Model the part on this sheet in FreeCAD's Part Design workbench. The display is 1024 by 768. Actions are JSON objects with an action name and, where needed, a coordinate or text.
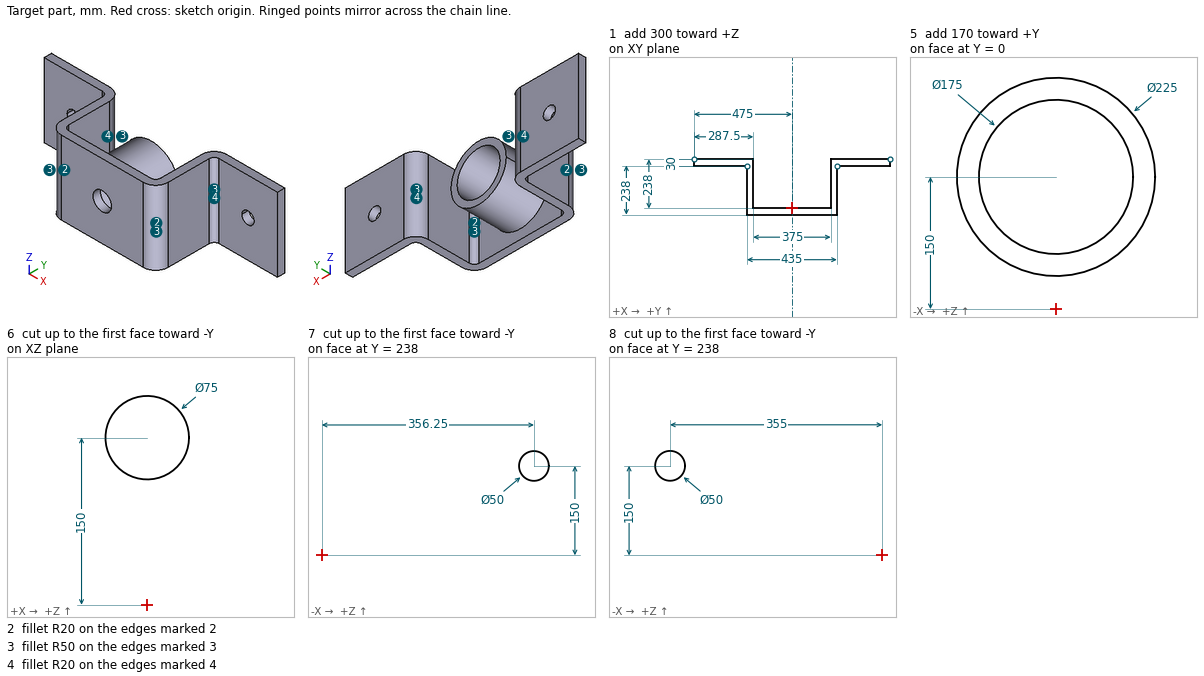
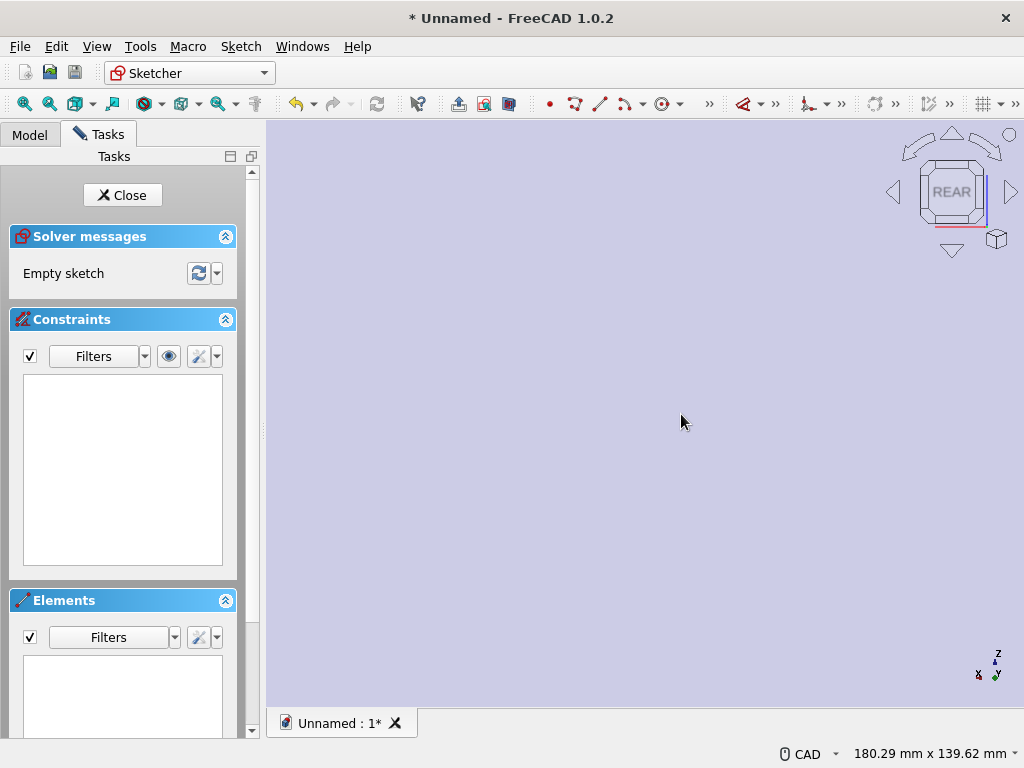
{"action": "scroll", "coordinate": [572, 399], "scroll_direction": "up", "scroll_amount": 3}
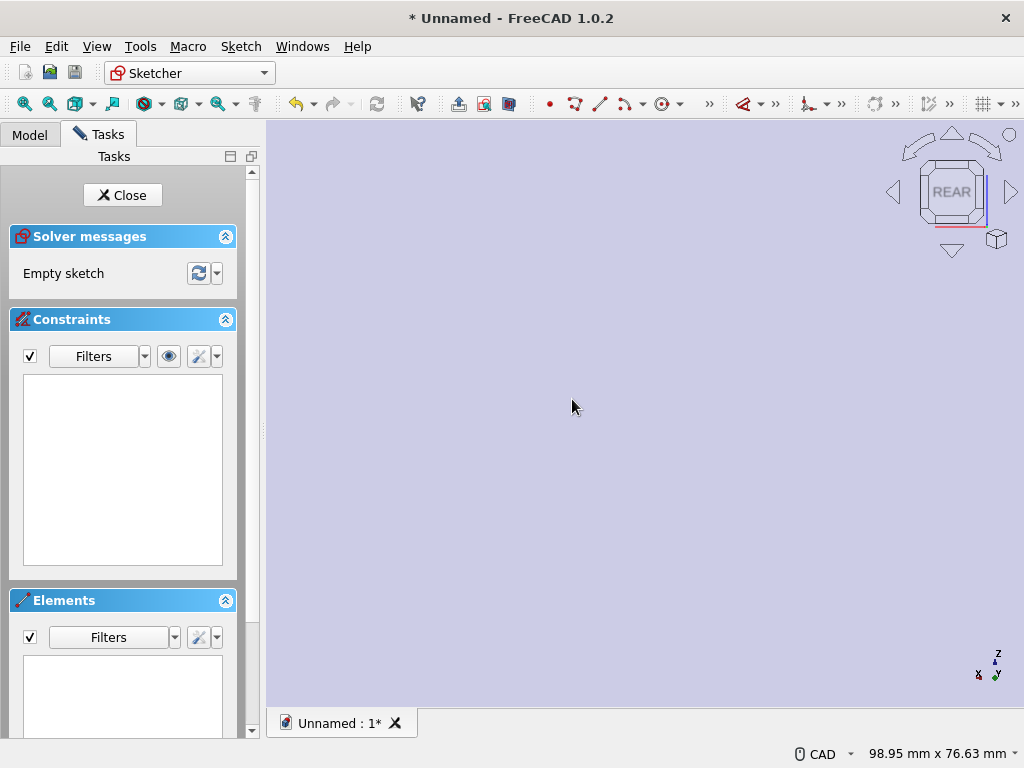
{"action": "left_click", "coordinate": [662, 104]}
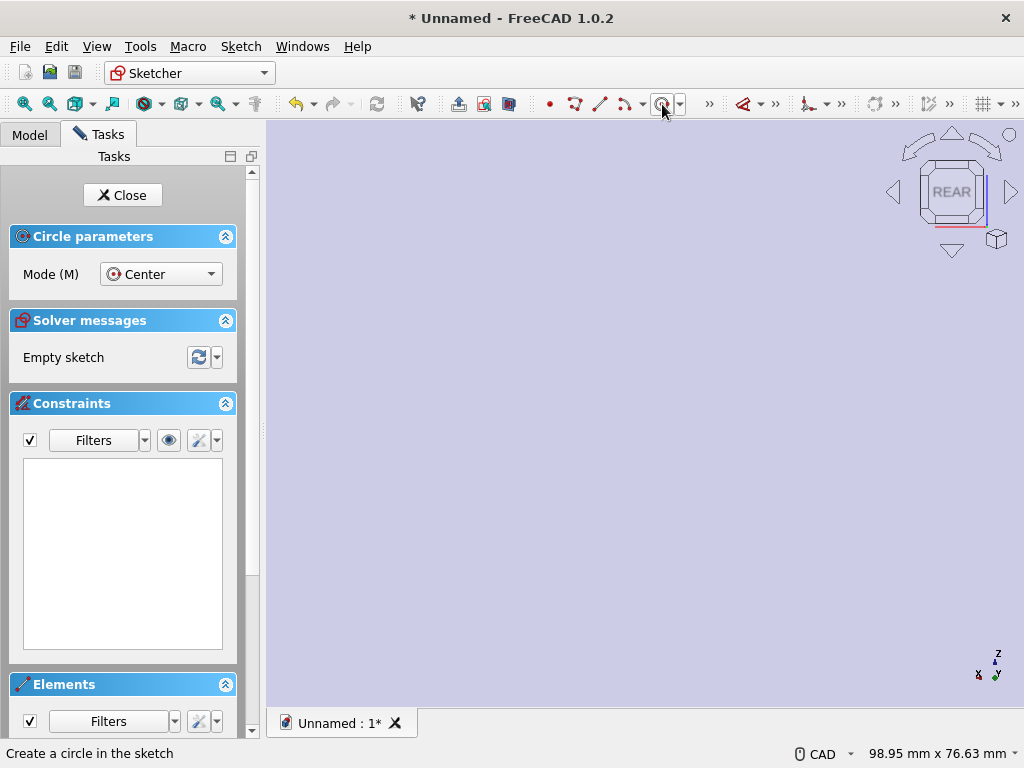
{"action": "left_click", "coordinate": [576, 413]}
{"action": "left_click", "coordinate": [711, 278]}
{"action": "key", "text": "Escape"}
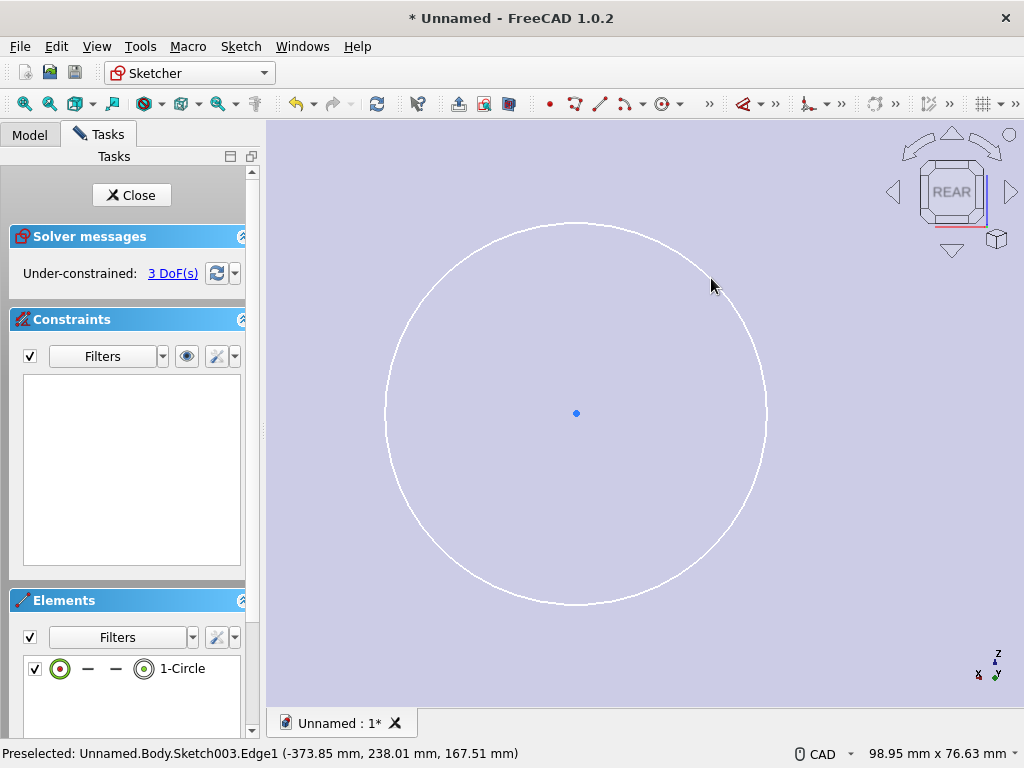
{"action": "left_click", "coordinate": [742, 104]}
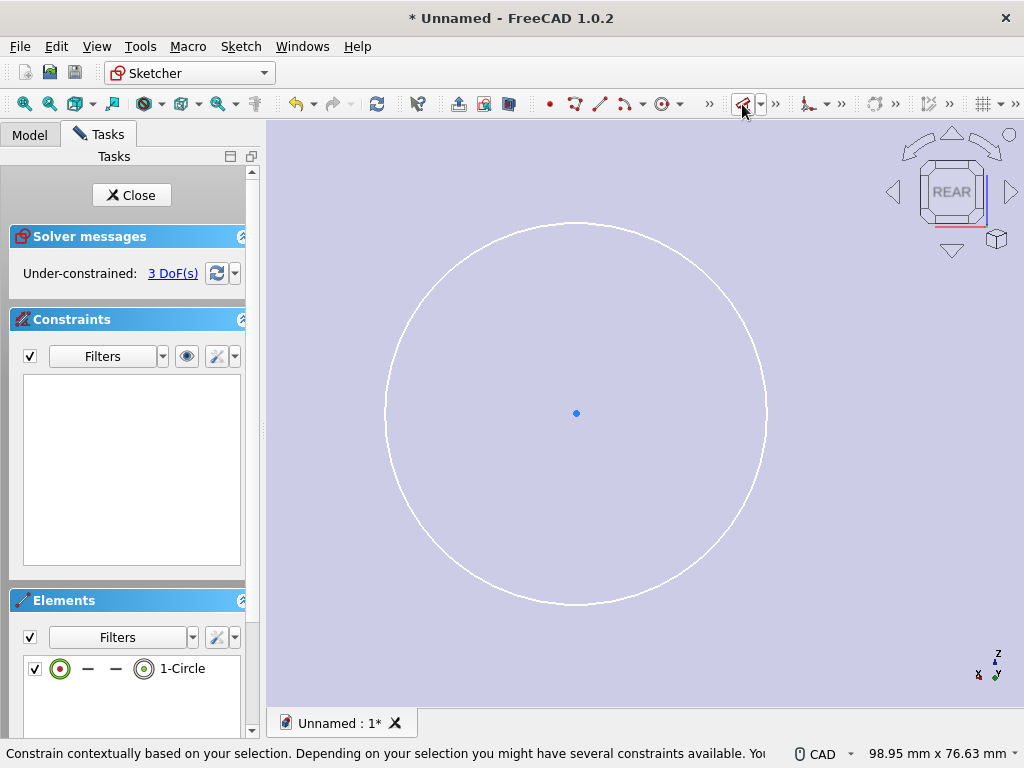
{"action": "left_click", "coordinate": [711, 279]}
{"action": "left_click", "coordinate": [734, 256]}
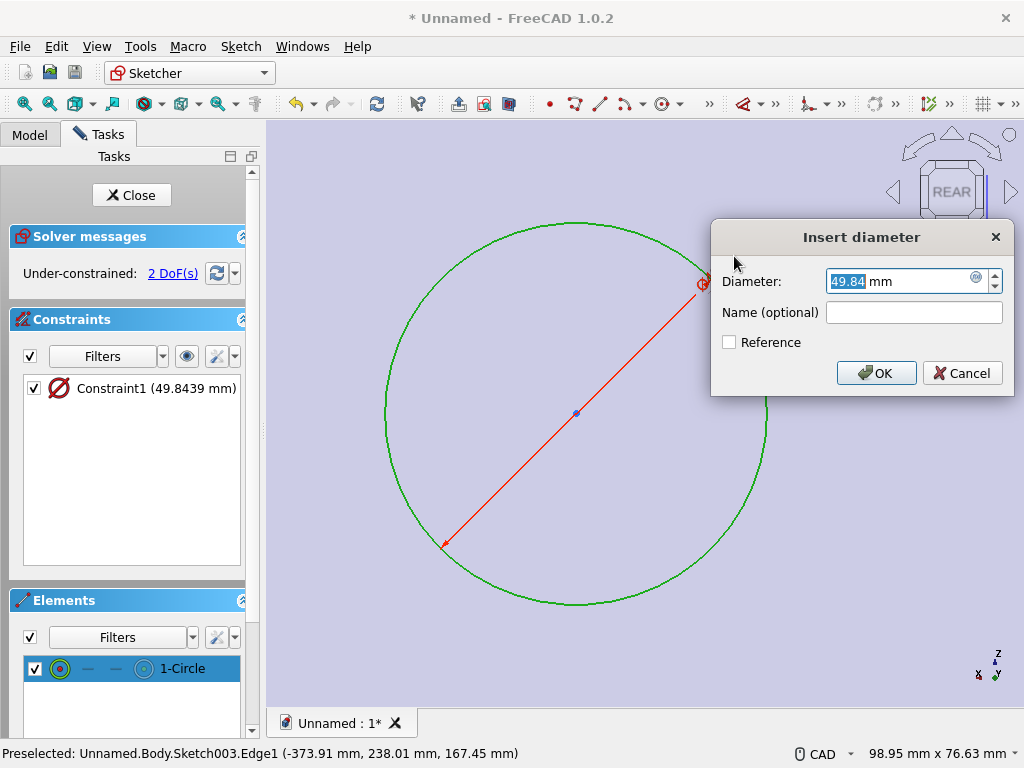
{"action": "type", "text": "50"}
{"action": "key", "text": "Return"}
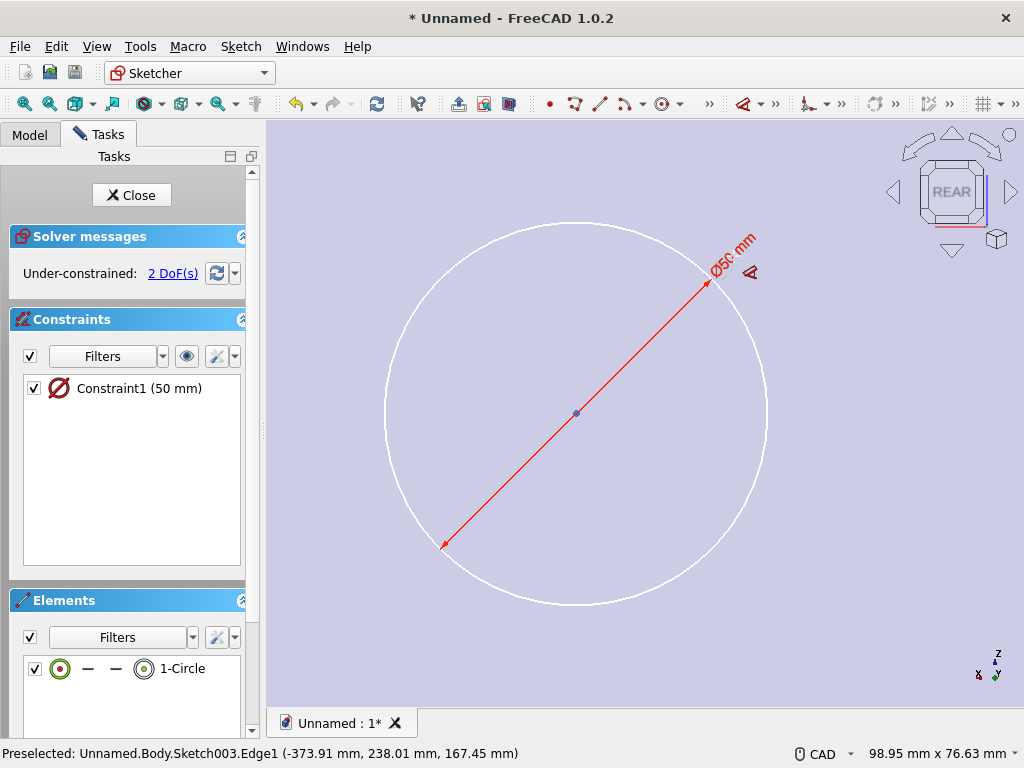
{"action": "left_click", "coordinate": [576, 414]}
{"action": "left_click", "coordinate": [610, 546]}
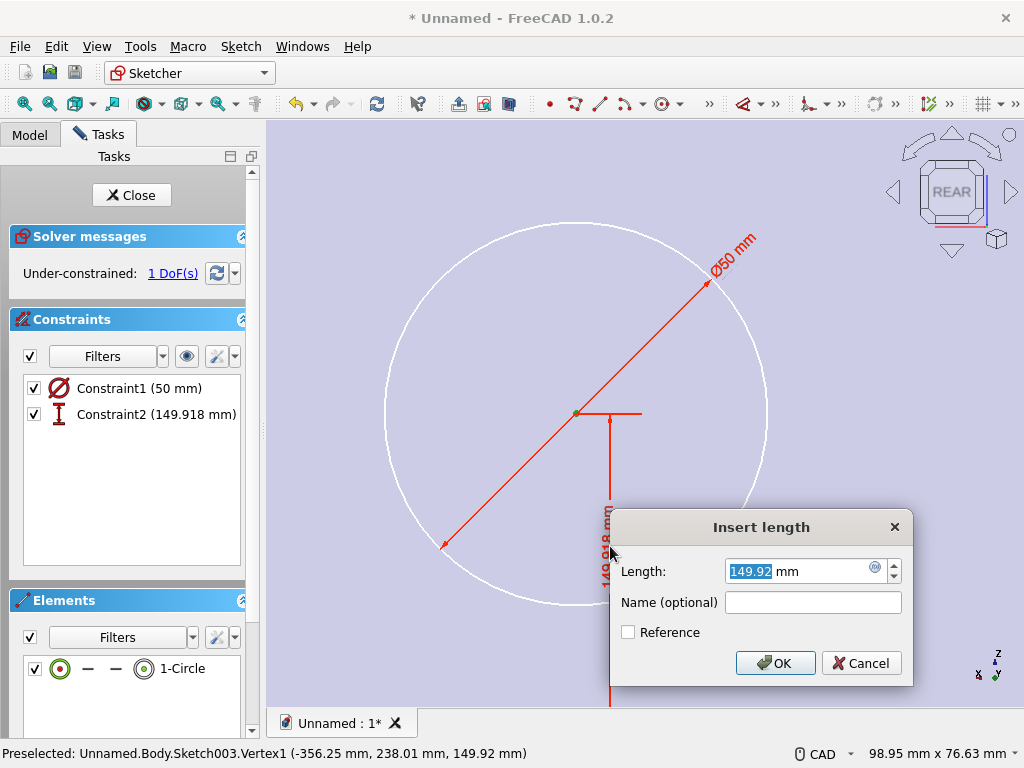
{"action": "type", "text": "150"}
{"action": "key", "text": "Return"}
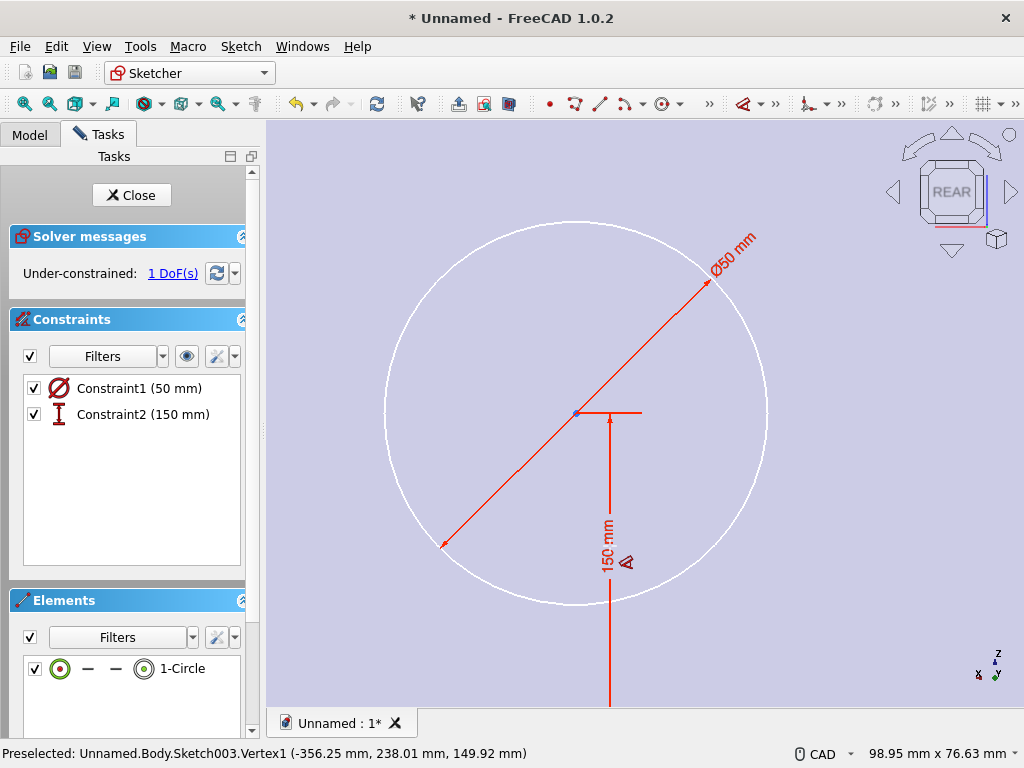
{"action": "left_click", "coordinate": [576, 413]}
{"action": "left_click", "coordinate": [435, 379]}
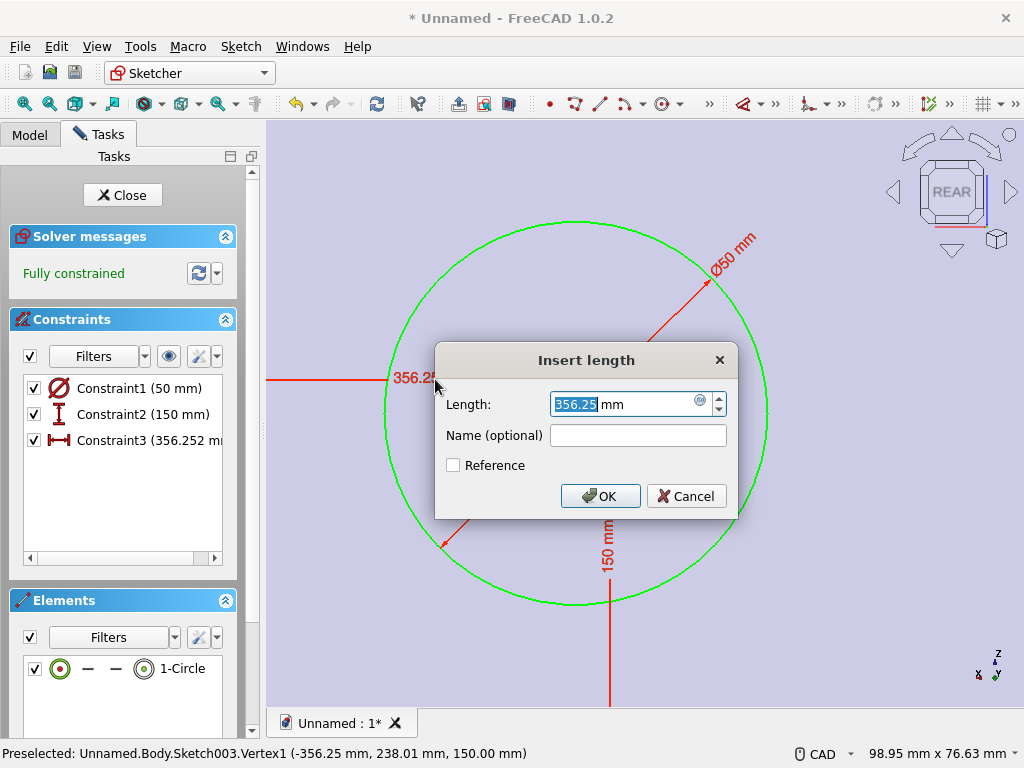
{"action": "type", "text": "356.25"}
{"action": "key", "text": "Return"}
{"action": "key", "text": "Escape"}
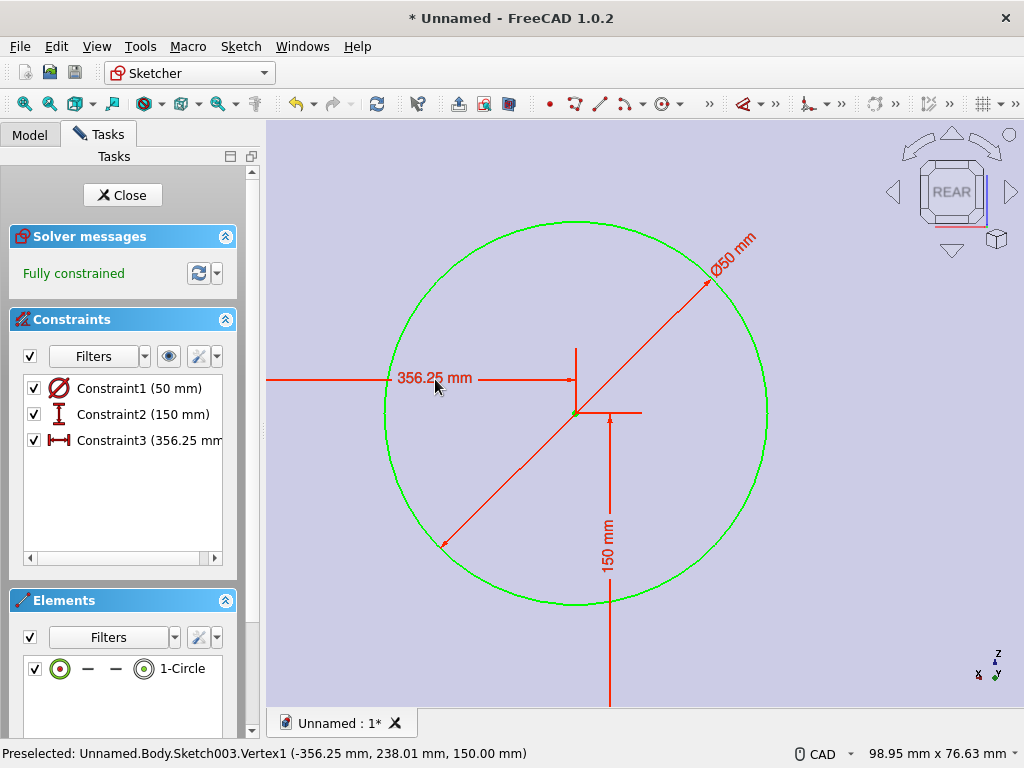
{"action": "left_click", "coordinate": [123, 195]}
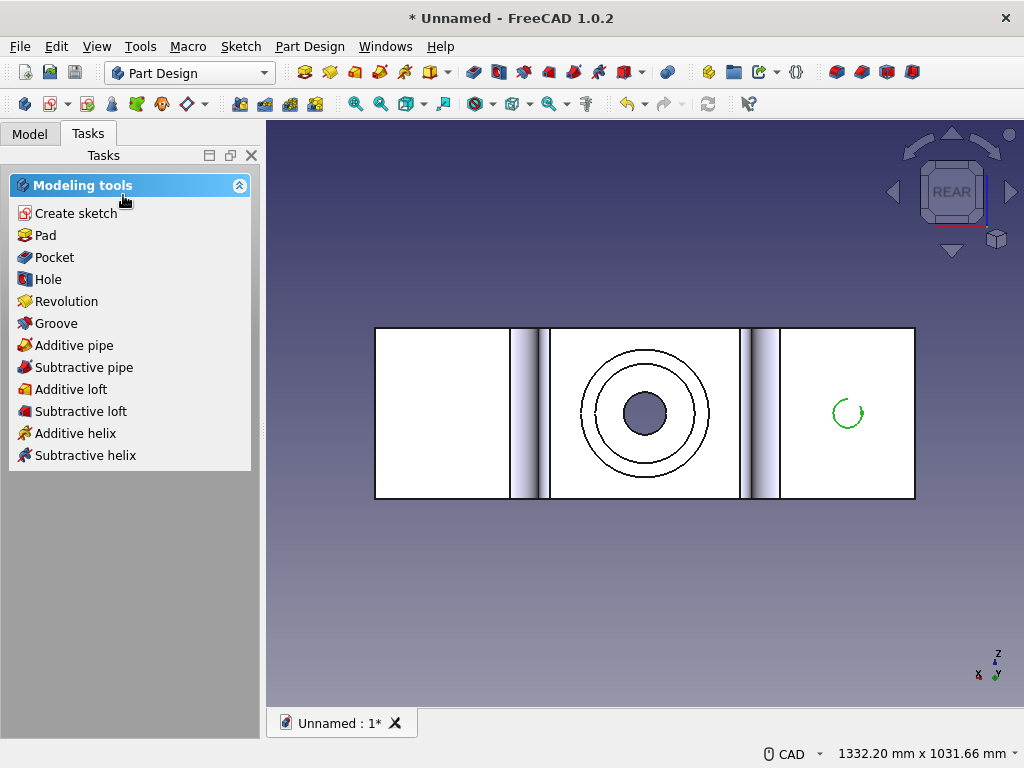
{"action": "left_click", "coordinate": [474, 72]}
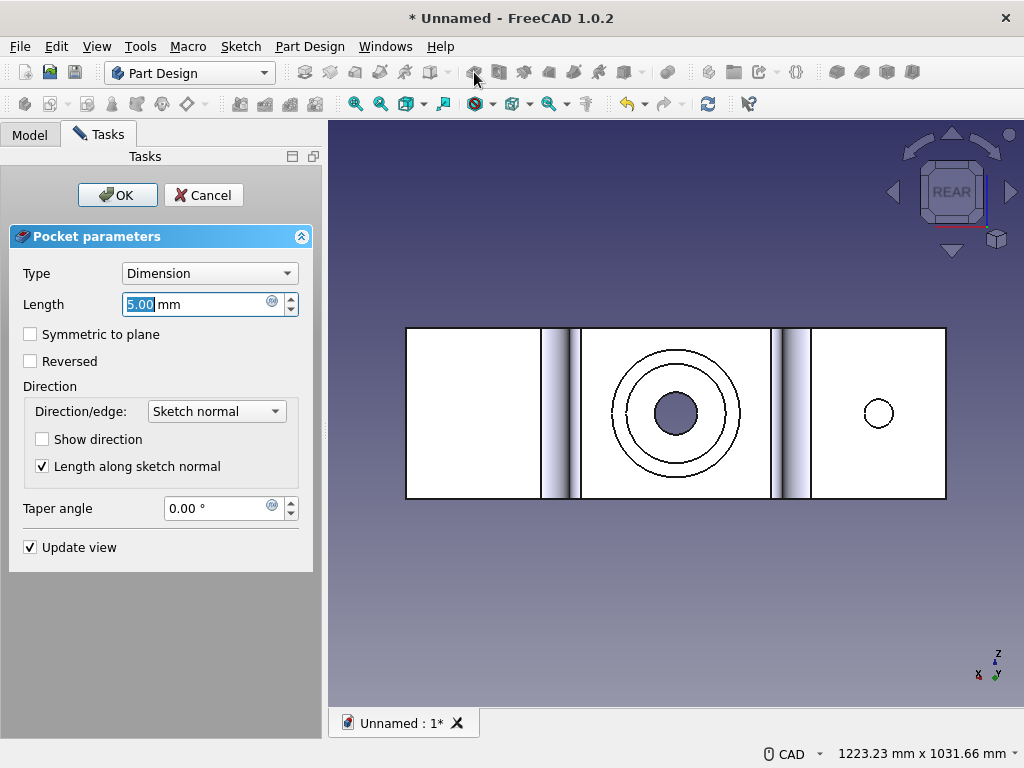
{"action": "left_click", "coordinate": [210, 274]}